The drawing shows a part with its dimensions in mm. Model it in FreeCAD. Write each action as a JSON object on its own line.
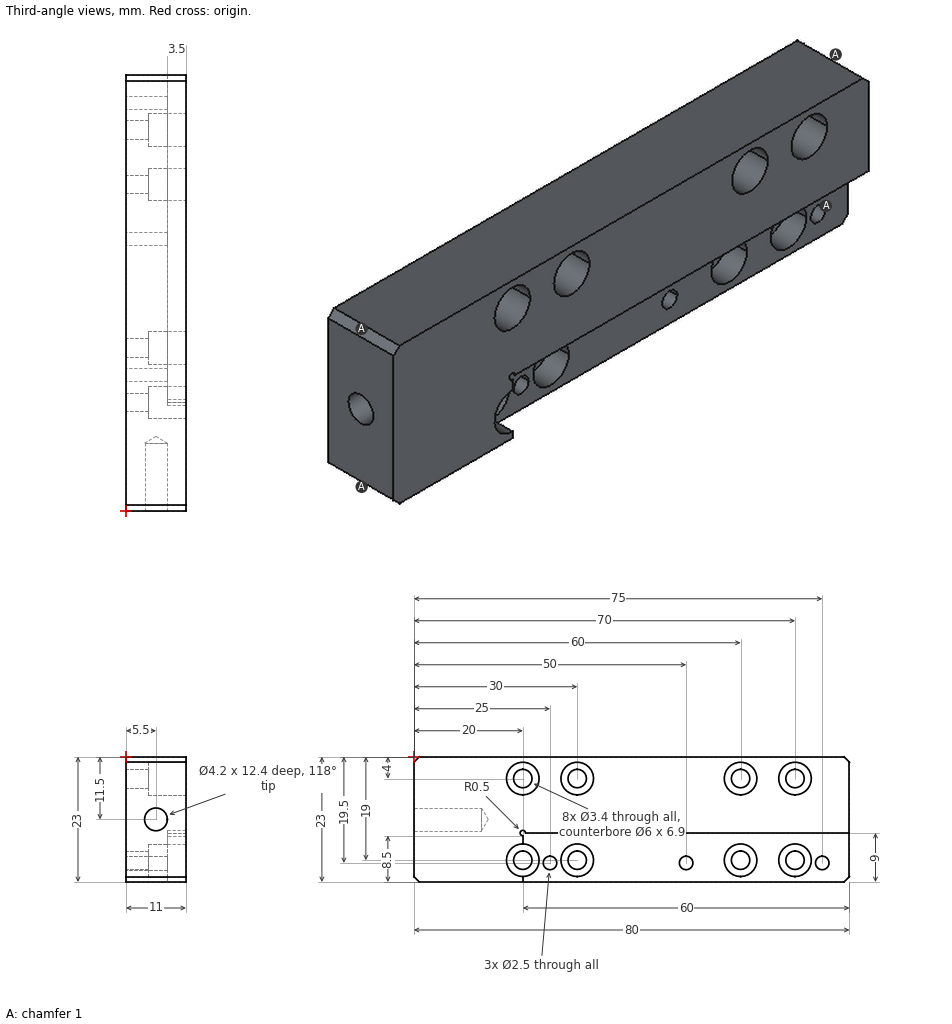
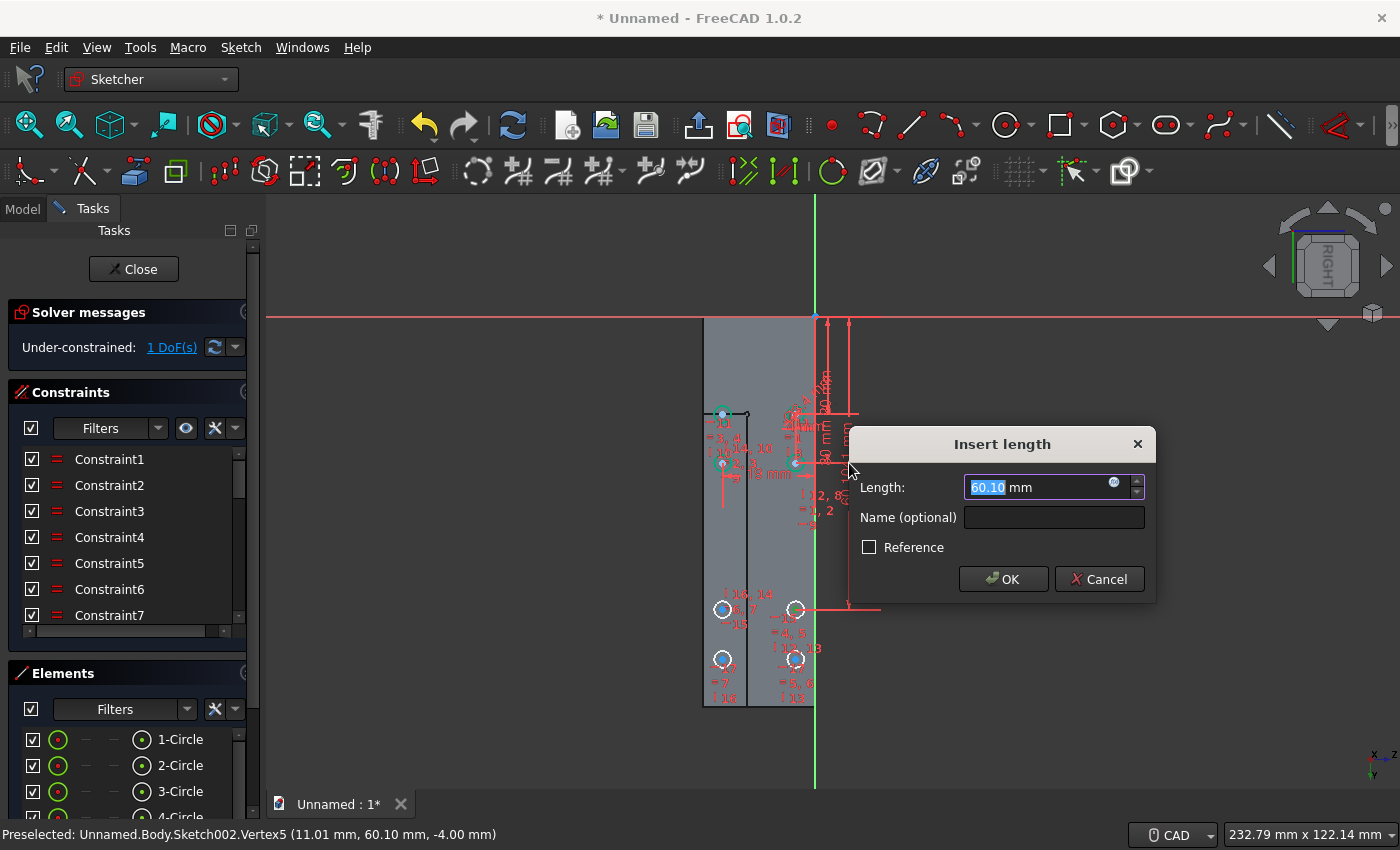
{"action": "type", "text": "60"}
{"action": "key", "text": "Return"}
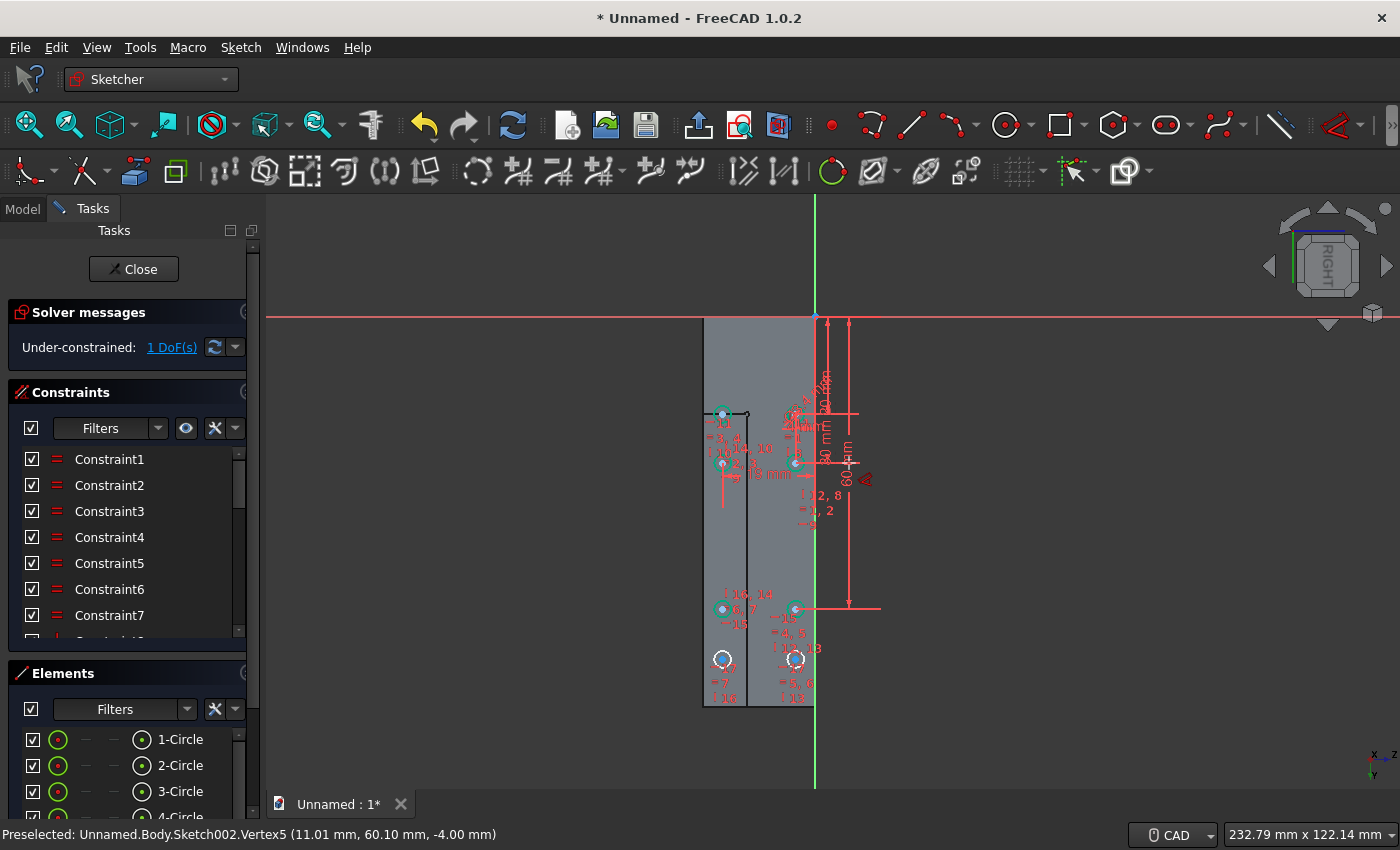
{"action": "left_click", "coordinate": [796, 659]}
{"action": "left_click", "coordinate": [849, 488]}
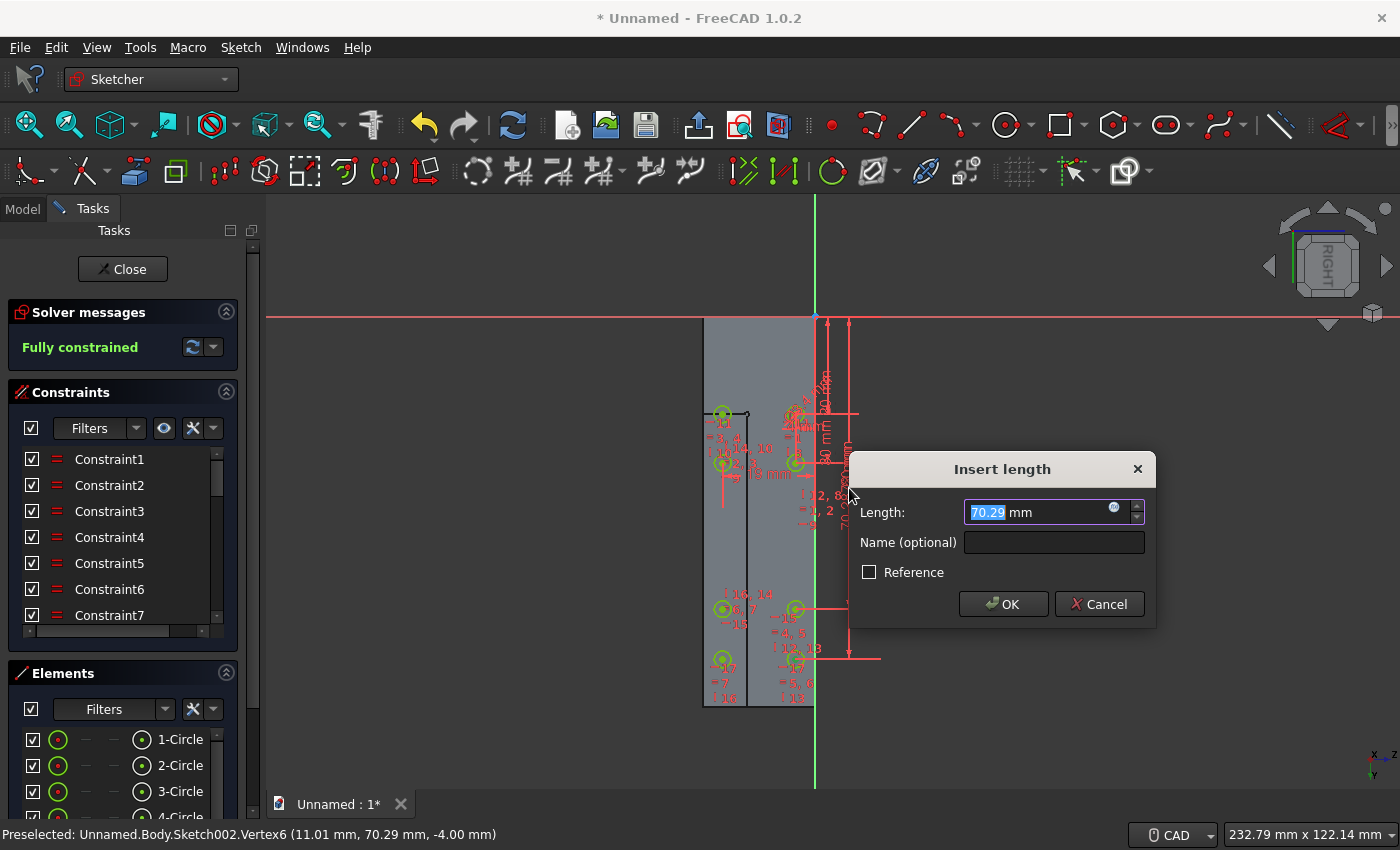
{"action": "type", "text": "70"}
{"action": "key", "text": "Return"}
{"action": "key", "text": "Escape"}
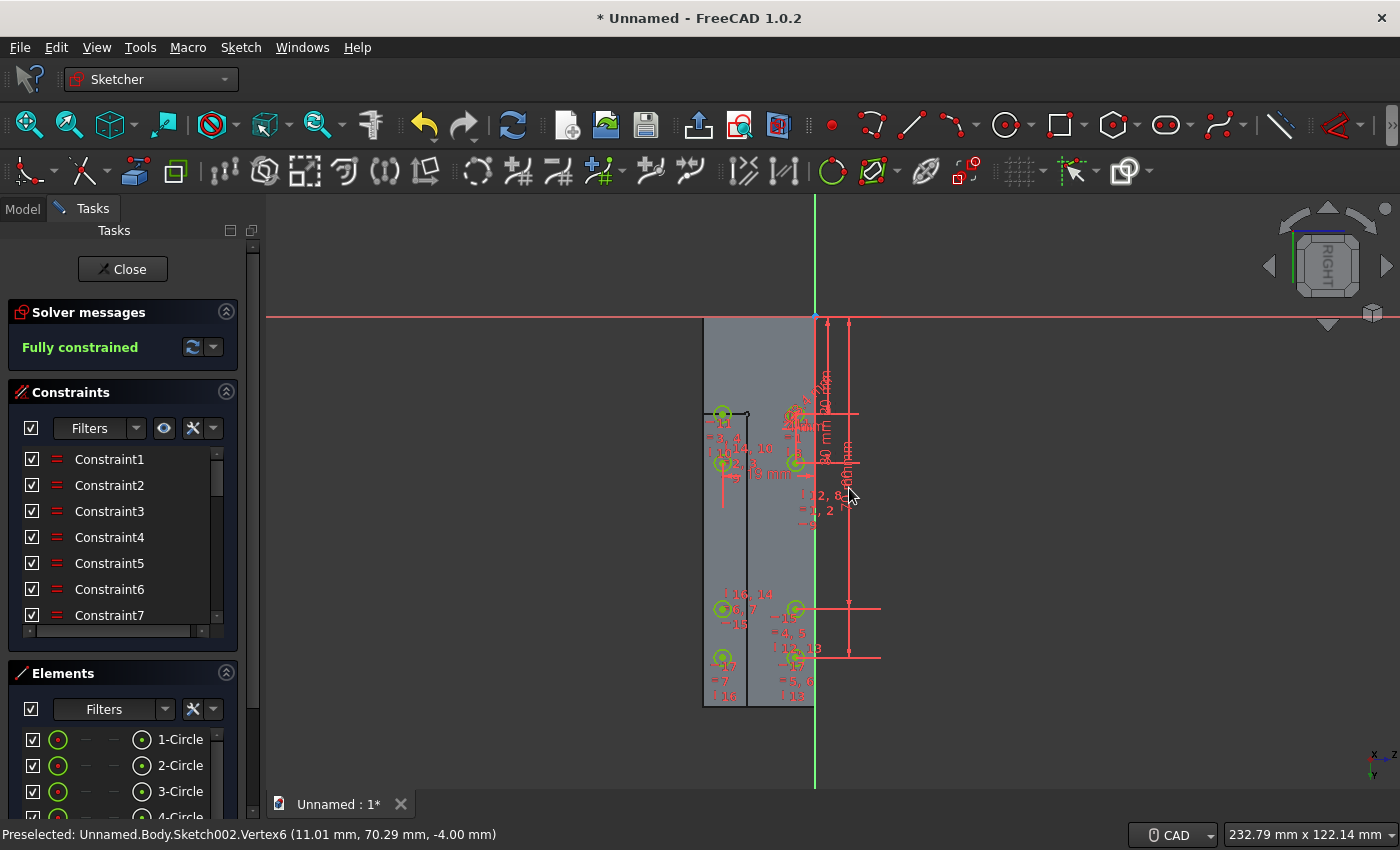
{"action": "left_click", "coordinate": [123, 269]}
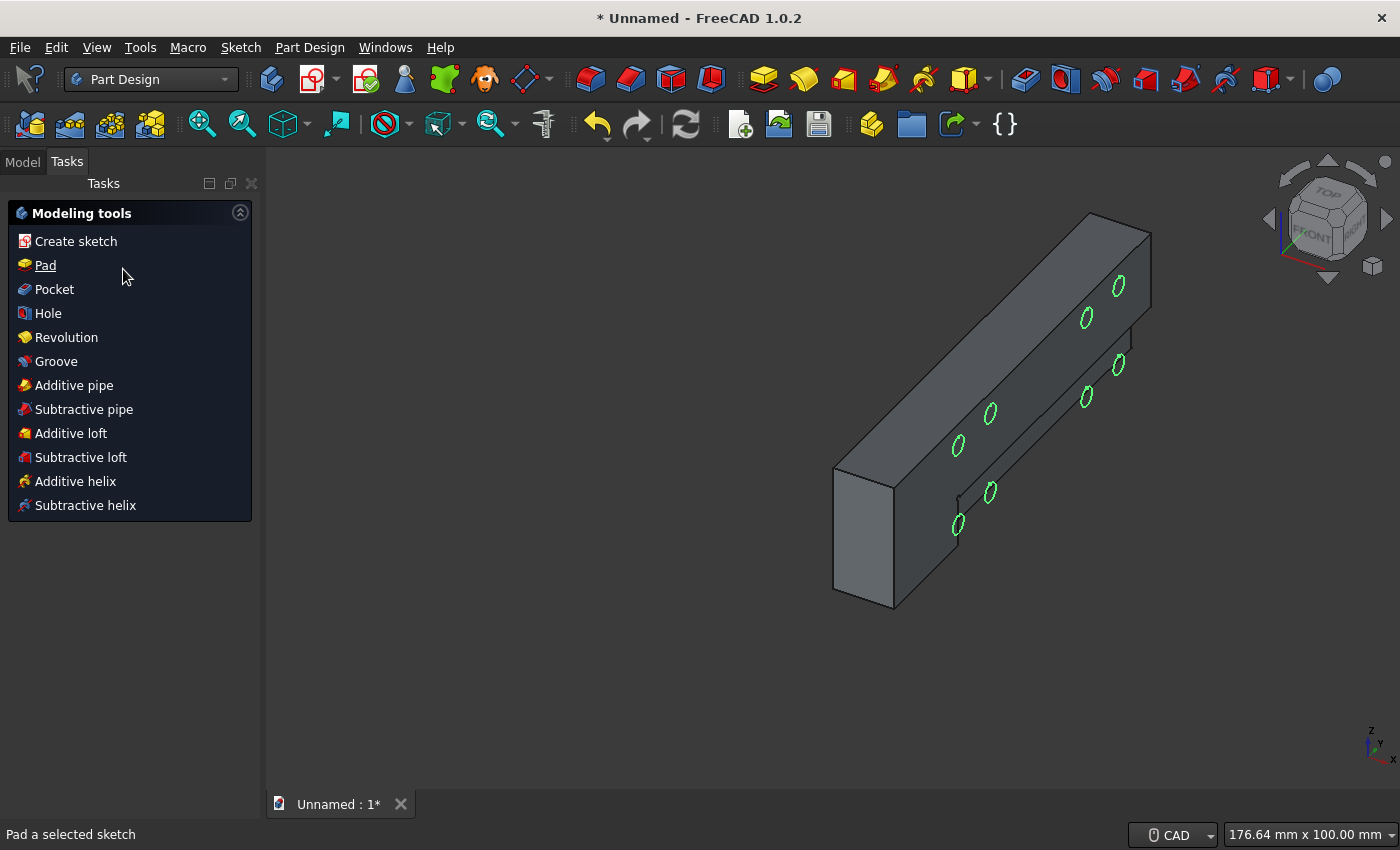
{"action": "left_click", "coordinate": [1066, 80]}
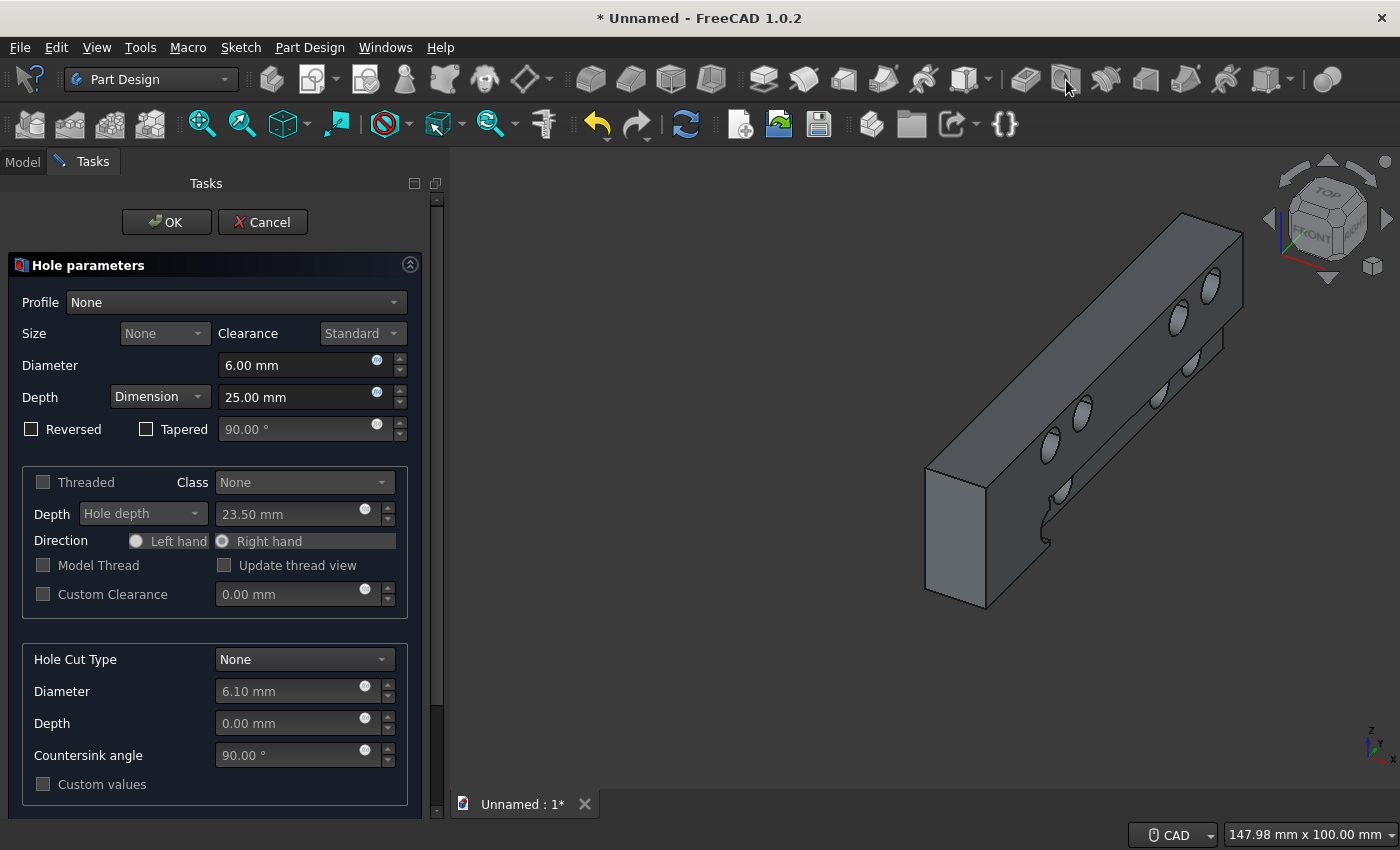
{"action": "triple_click", "coordinate": [305, 365]}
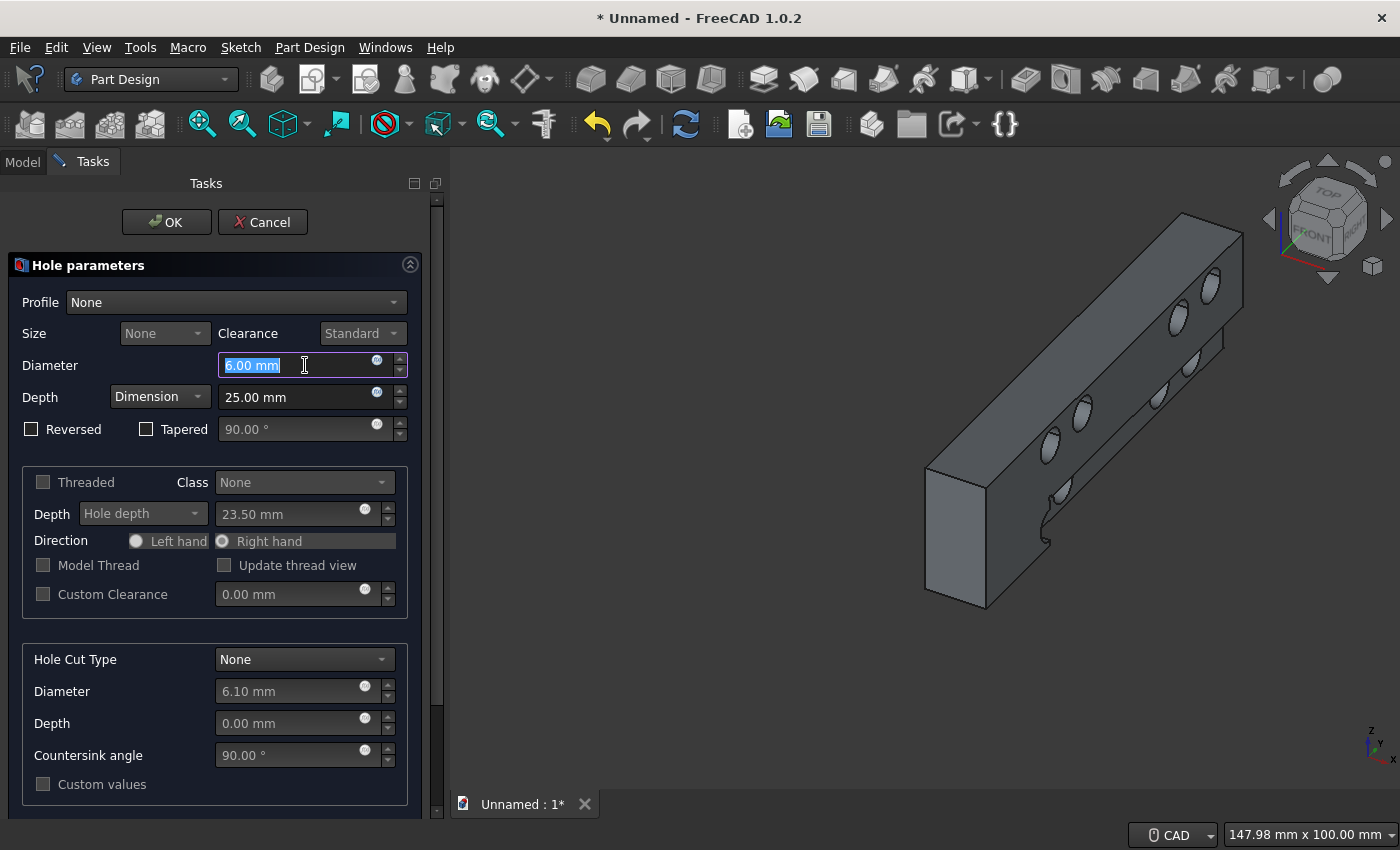
{"action": "type", "text": "3.4"}
{"action": "key", "text": "Tab"}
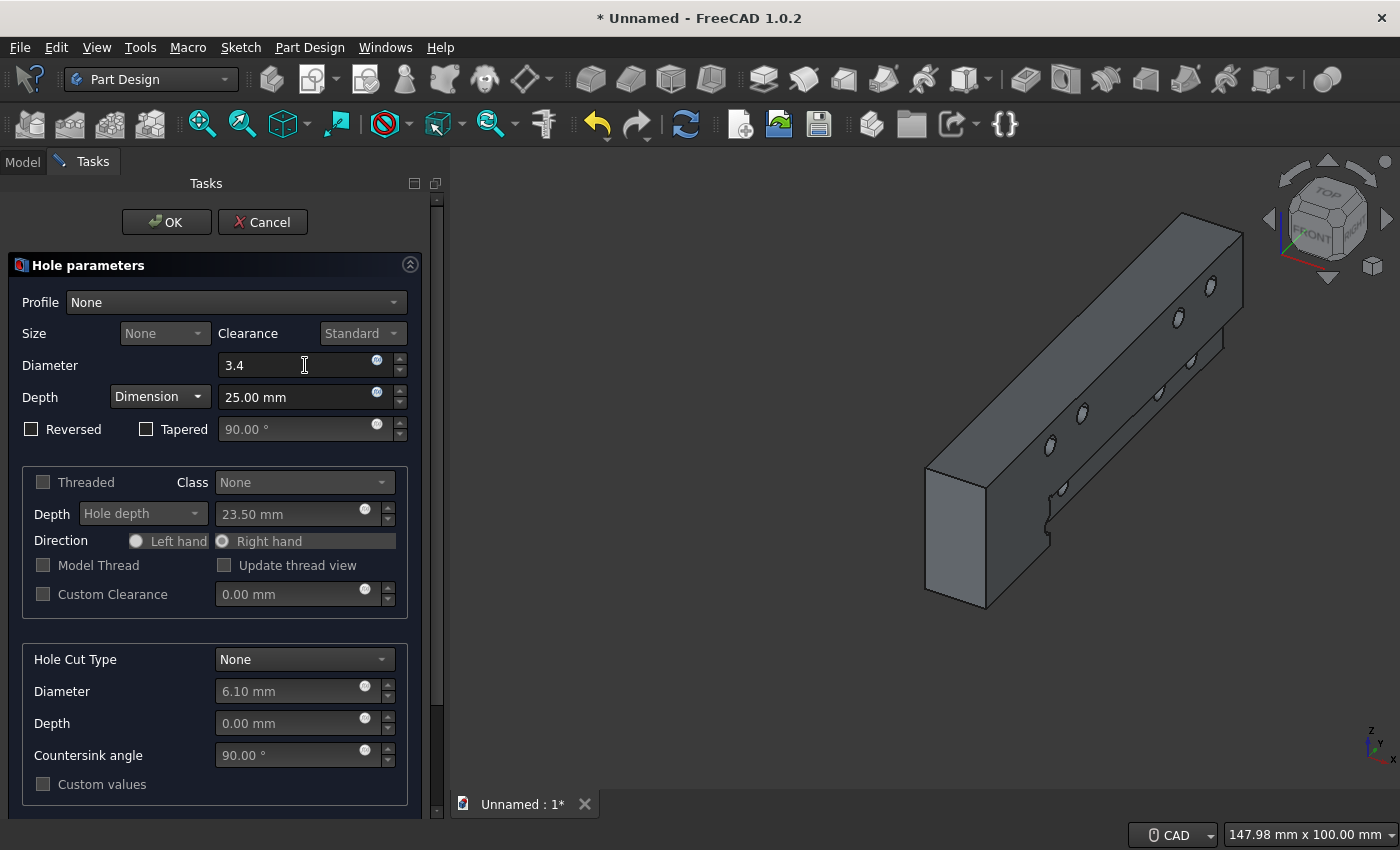
{"action": "left_click", "coordinate": [161, 396]}